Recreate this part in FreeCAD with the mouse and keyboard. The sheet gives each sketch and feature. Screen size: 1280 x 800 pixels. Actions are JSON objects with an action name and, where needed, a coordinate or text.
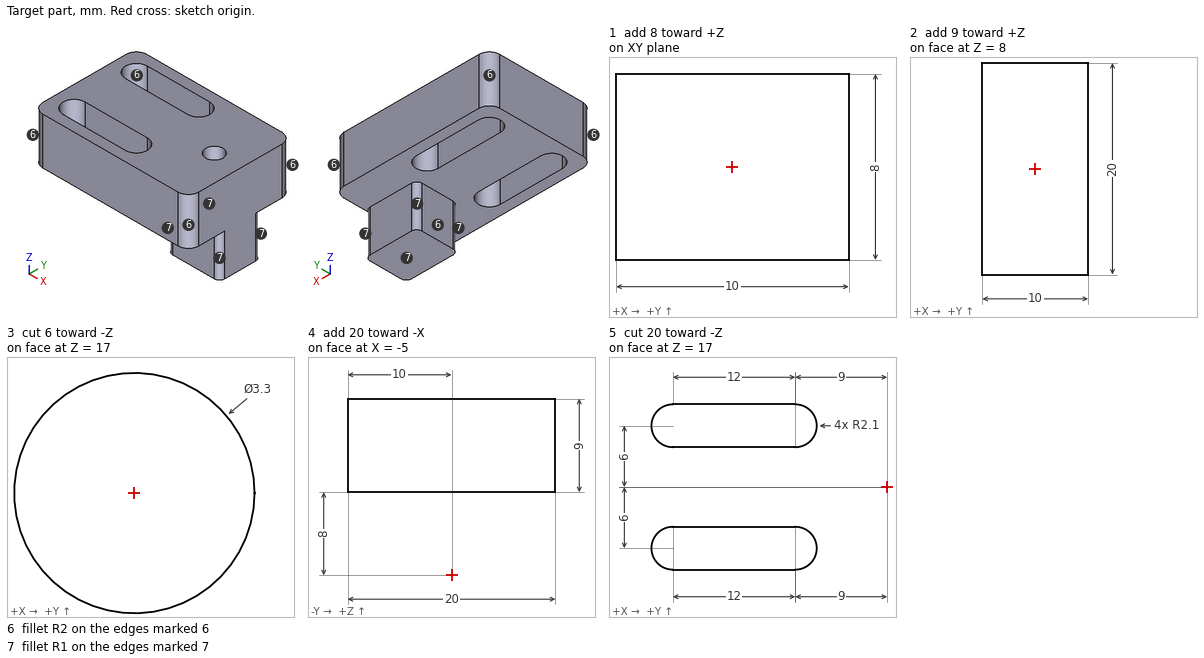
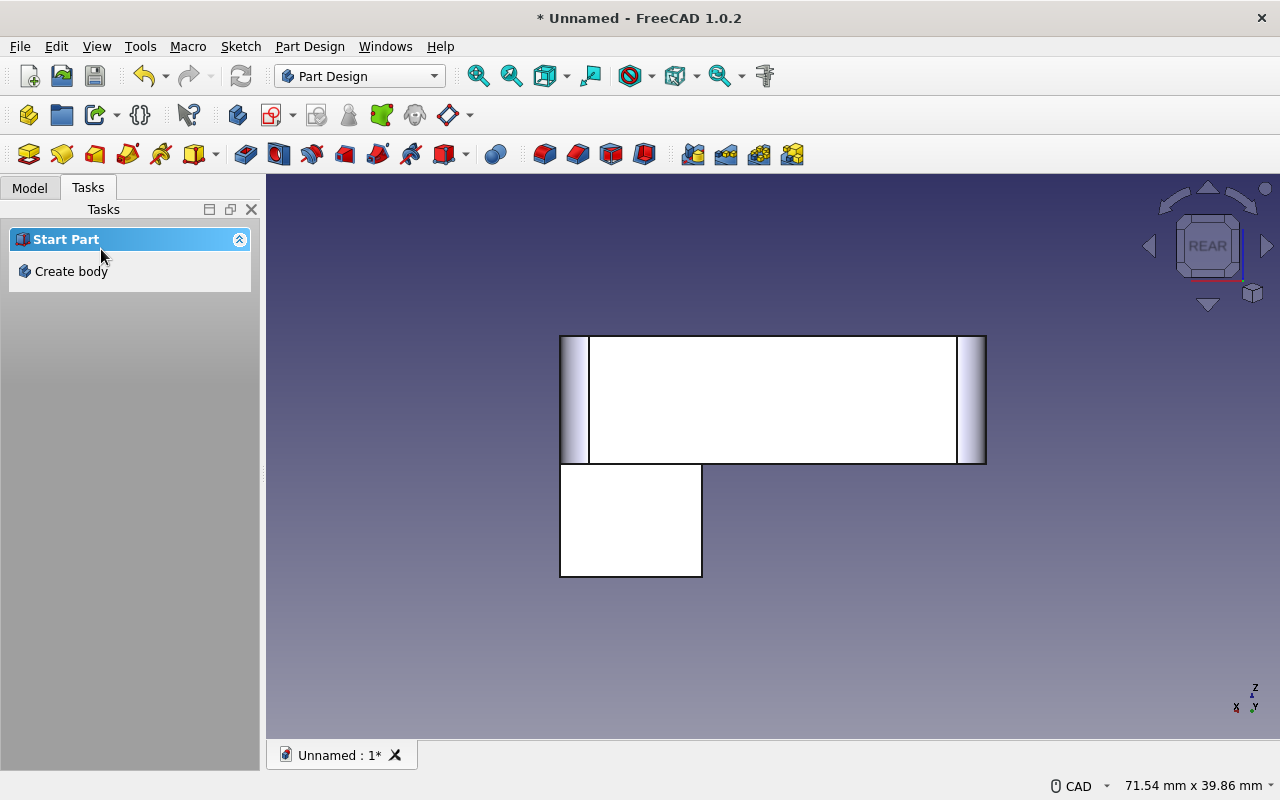
{"action": "left_click", "coordinate": [479, 76]}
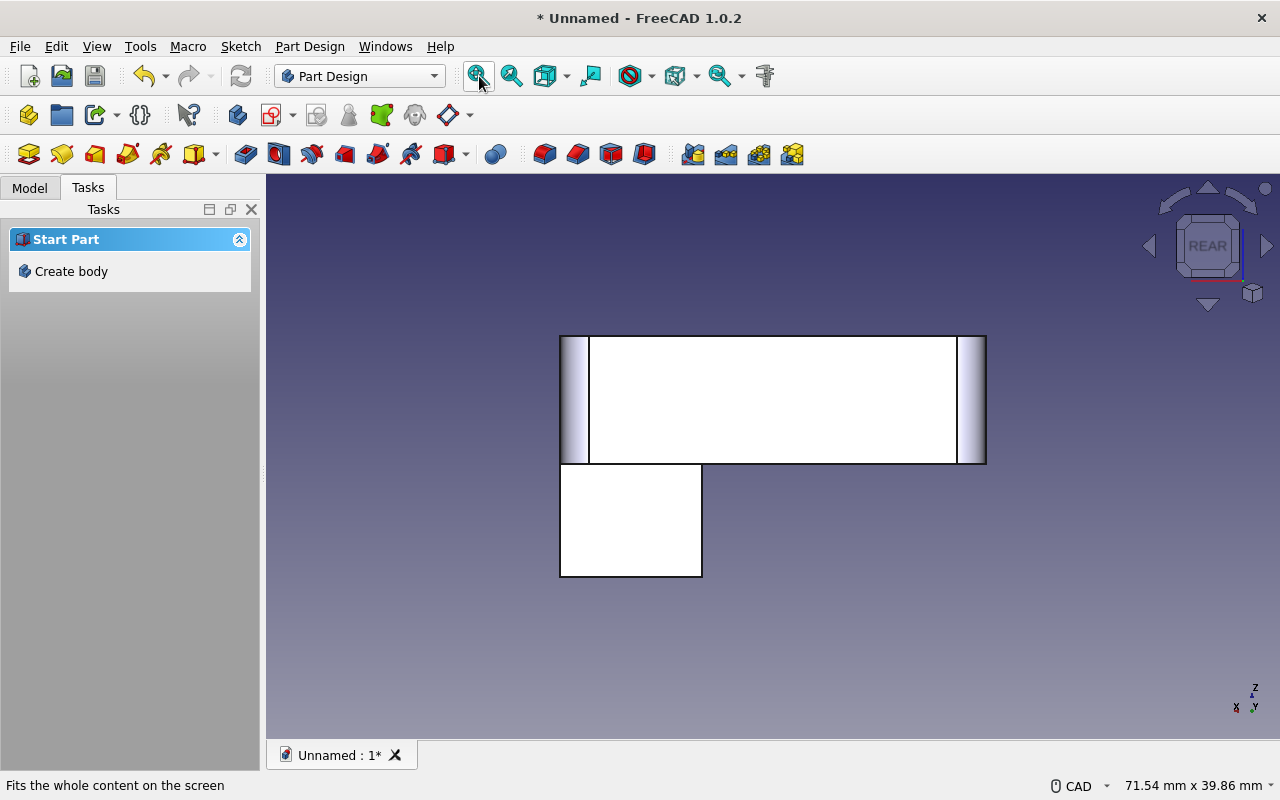
{"action": "left_click", "coordinate": [702, 519]}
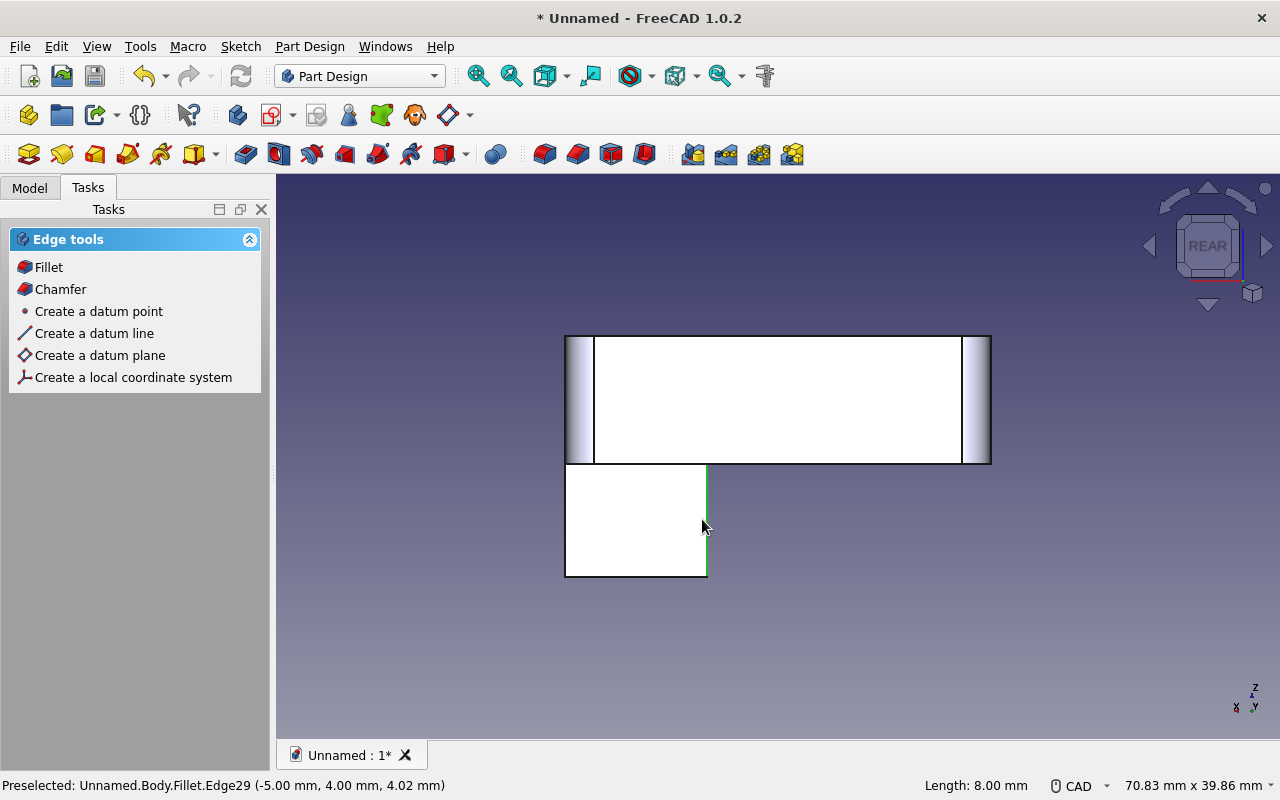
{"action": "left_click", "coordinate": [565, 519], "text": "ctrl"}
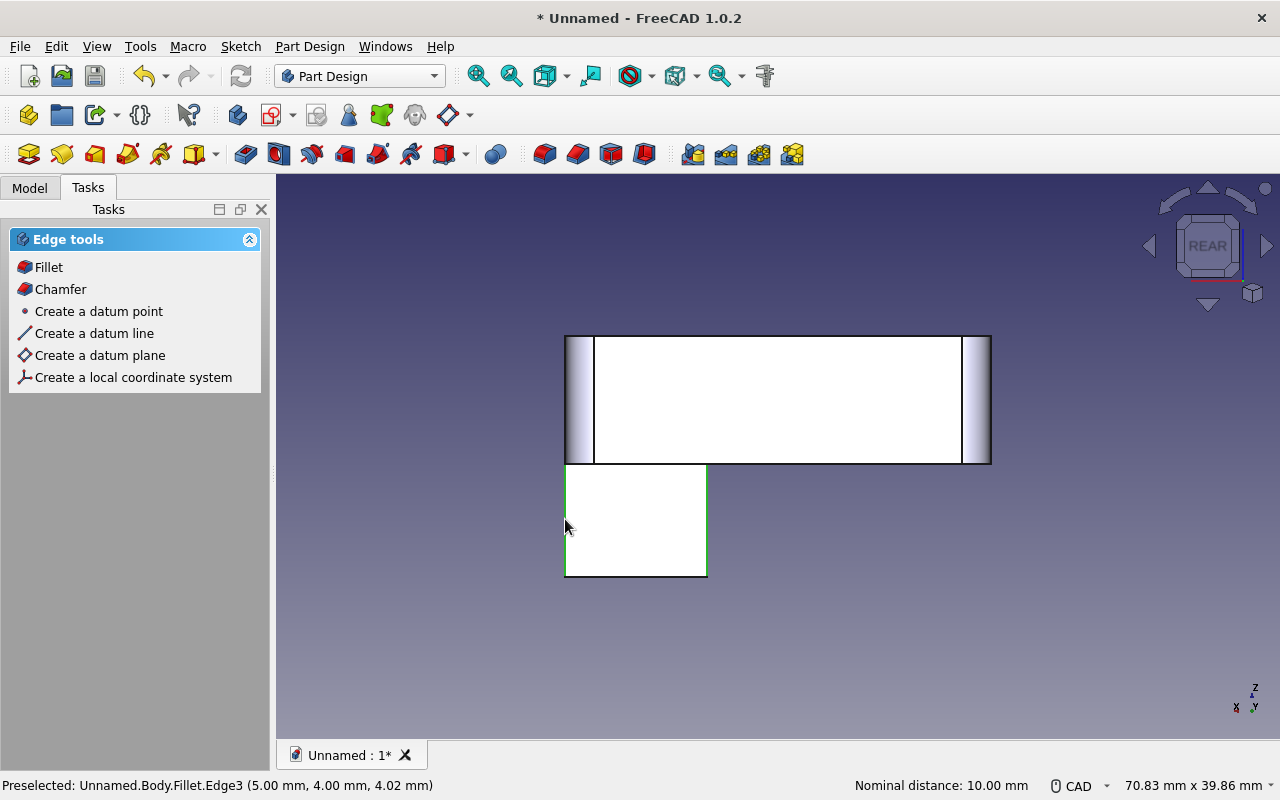
{"action": "key", "text": "0"}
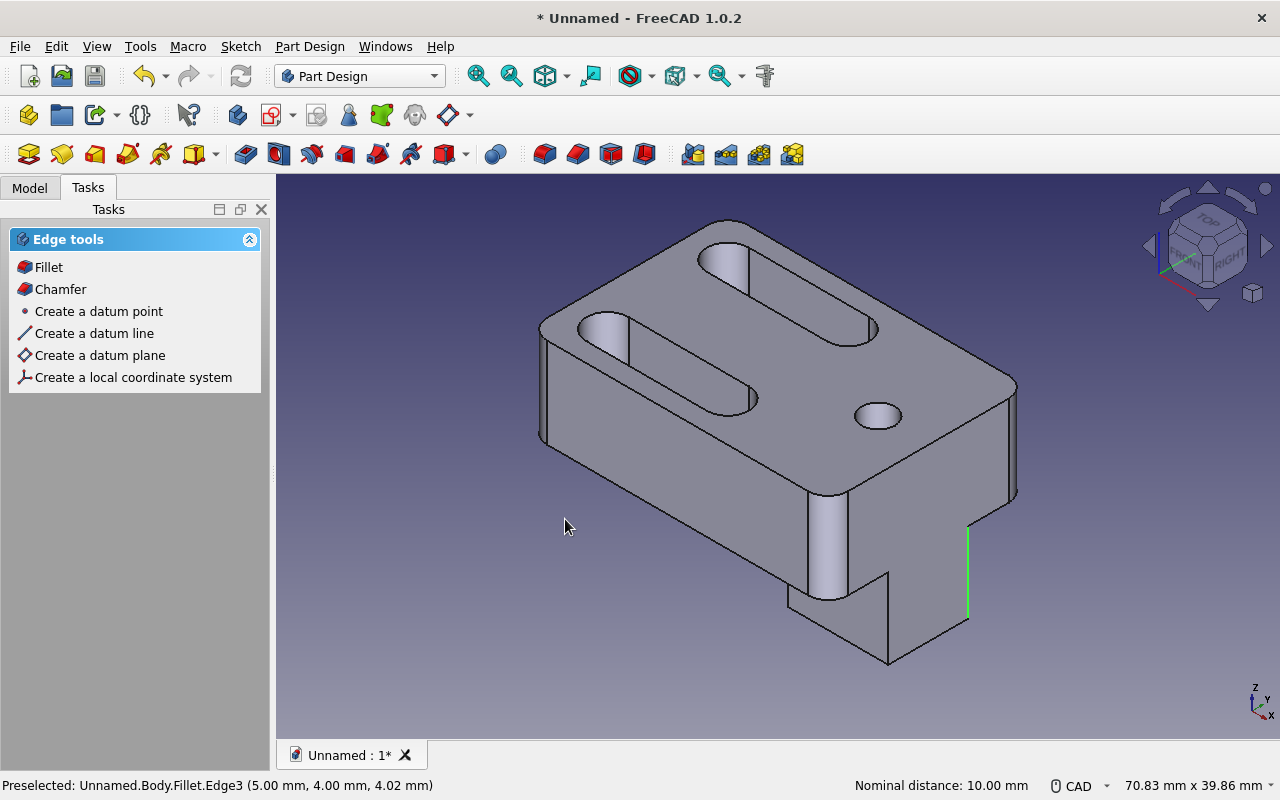
{"action": "left_click", "coordinate": [888, 618], "text": "ctrl"}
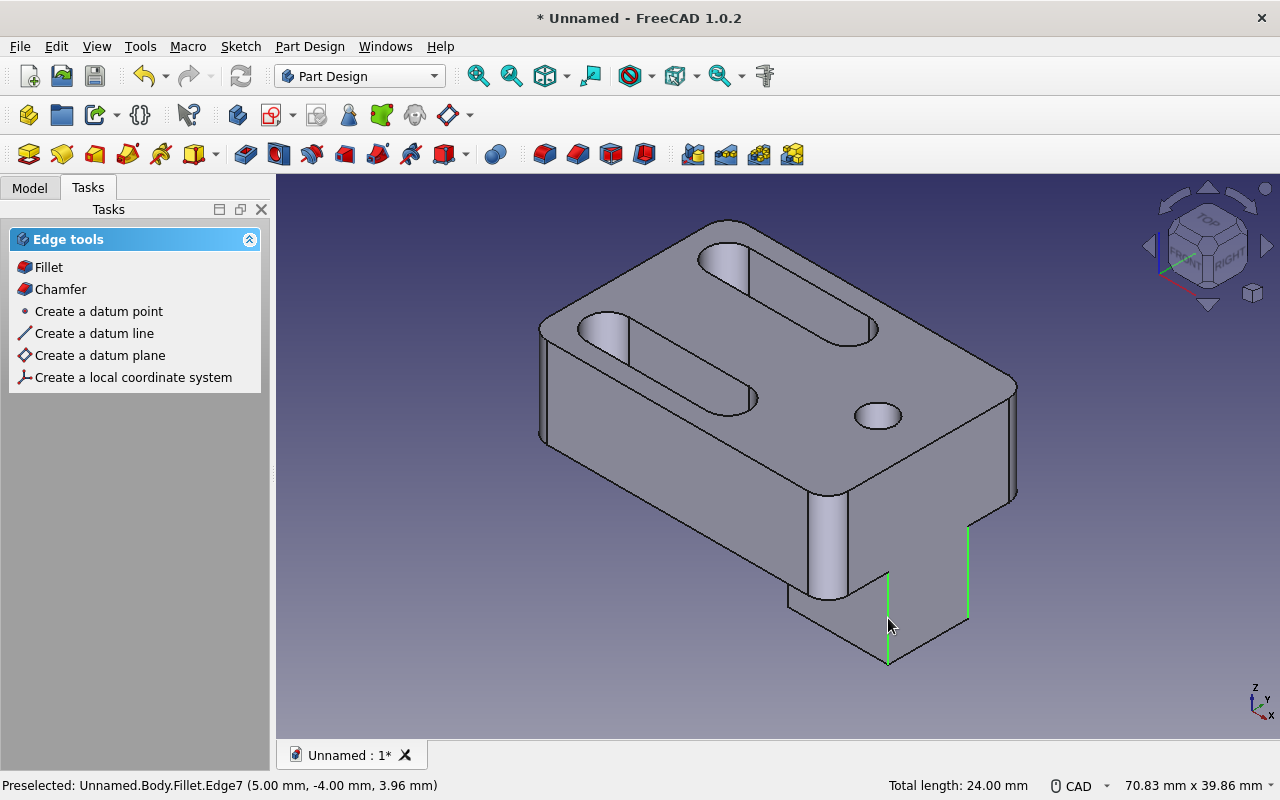
{"action": "key", "text": "2"}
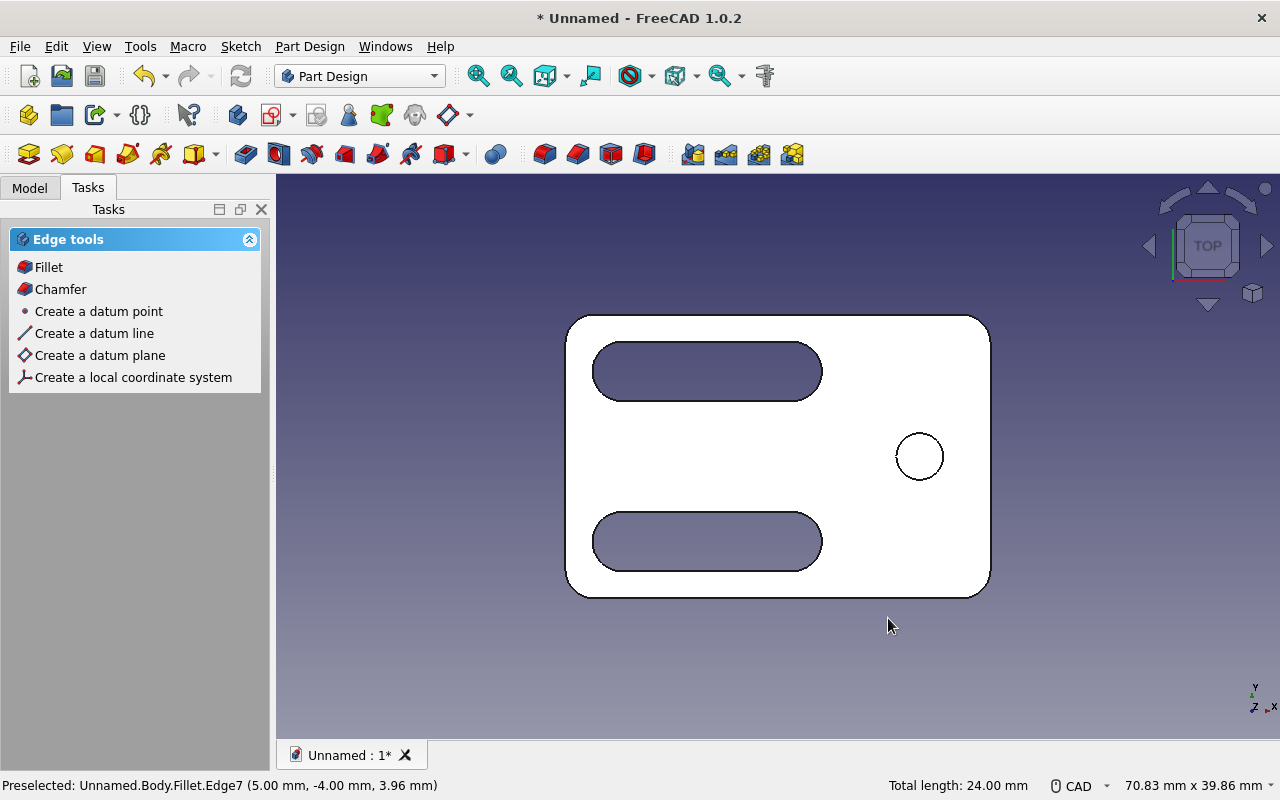
{"action": "key", "text": "1"}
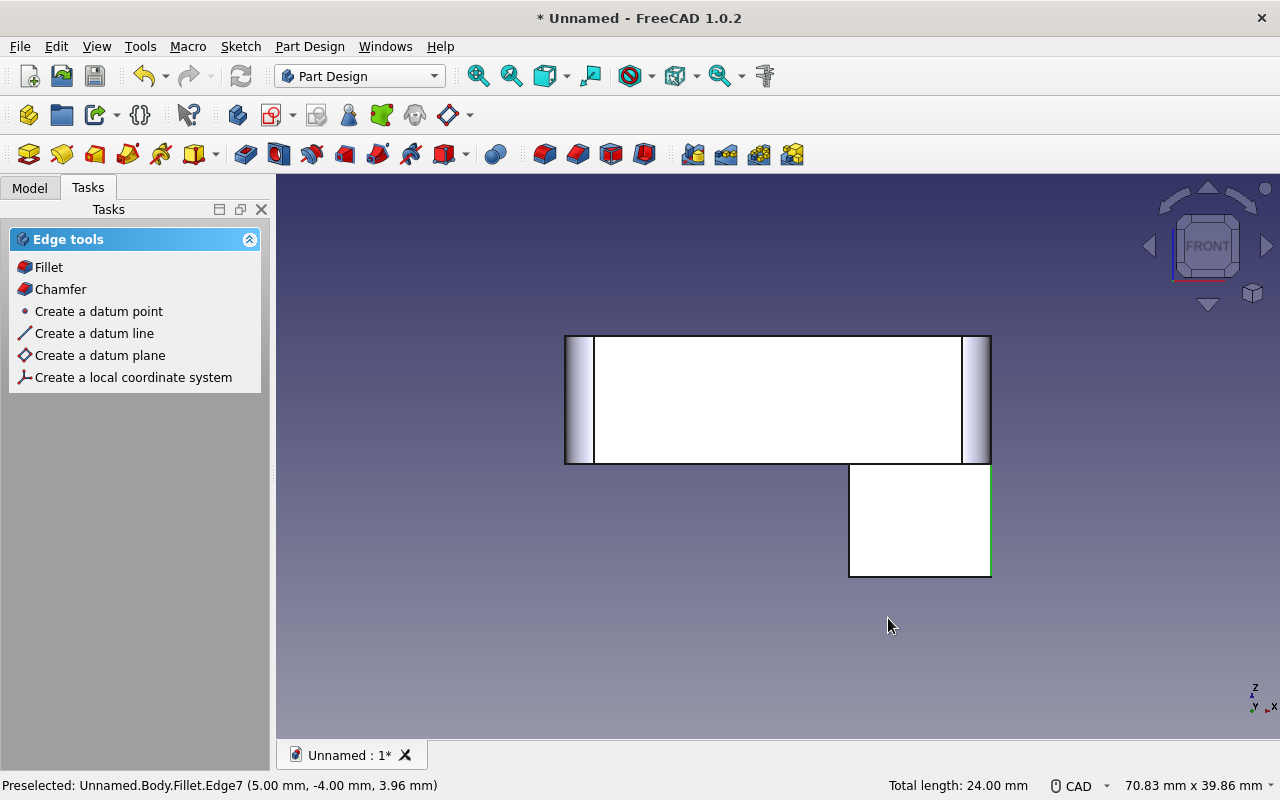
{"action": "key", "text": "v f"}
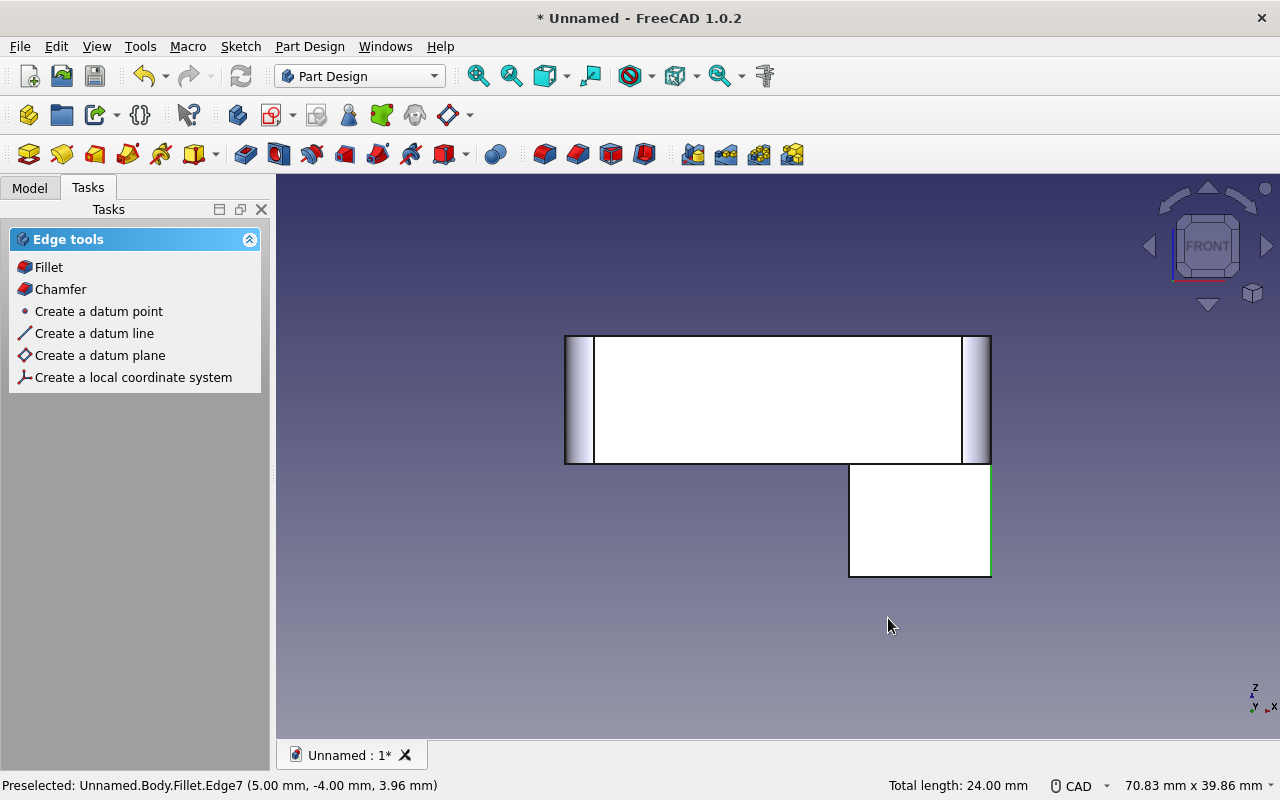
{"action": "left_click", "coordinate": [849, 519], "text": "ctrl"}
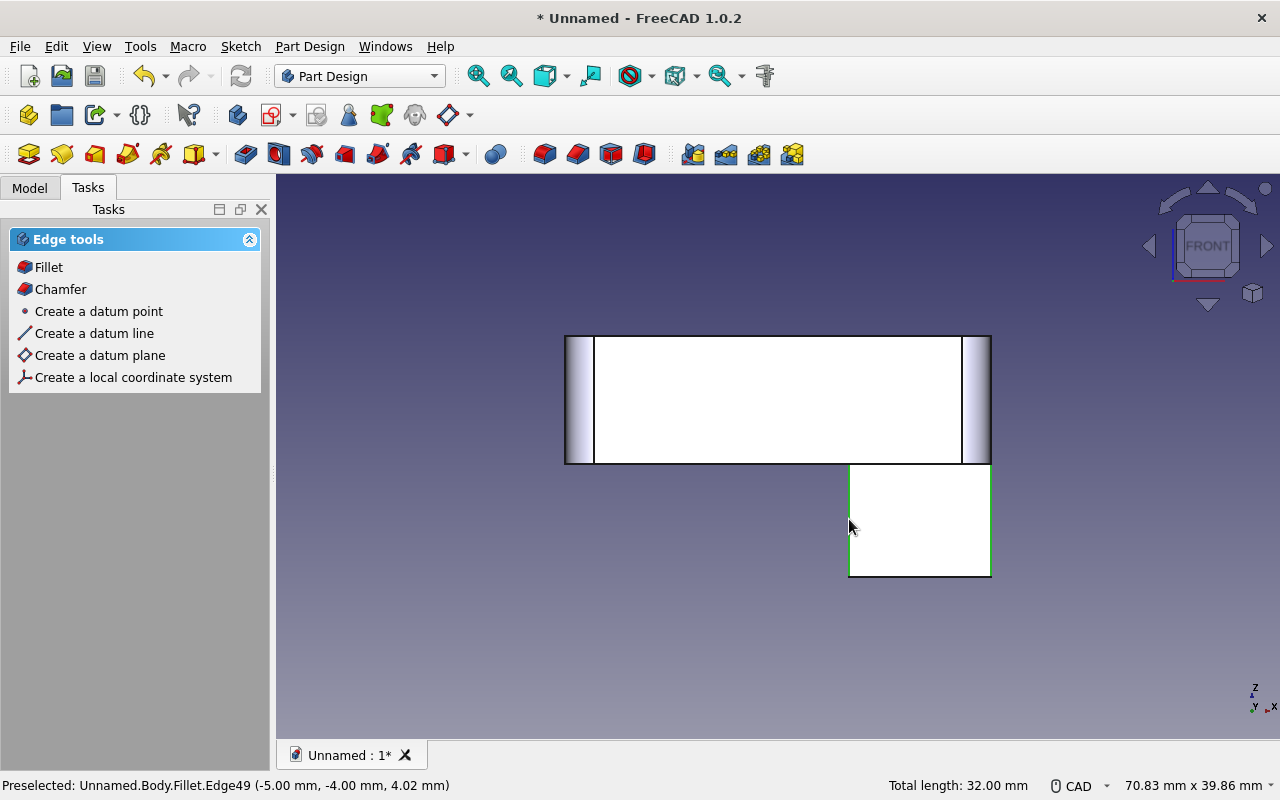
{"action": "left_click", "coordinate": [545, 154]}